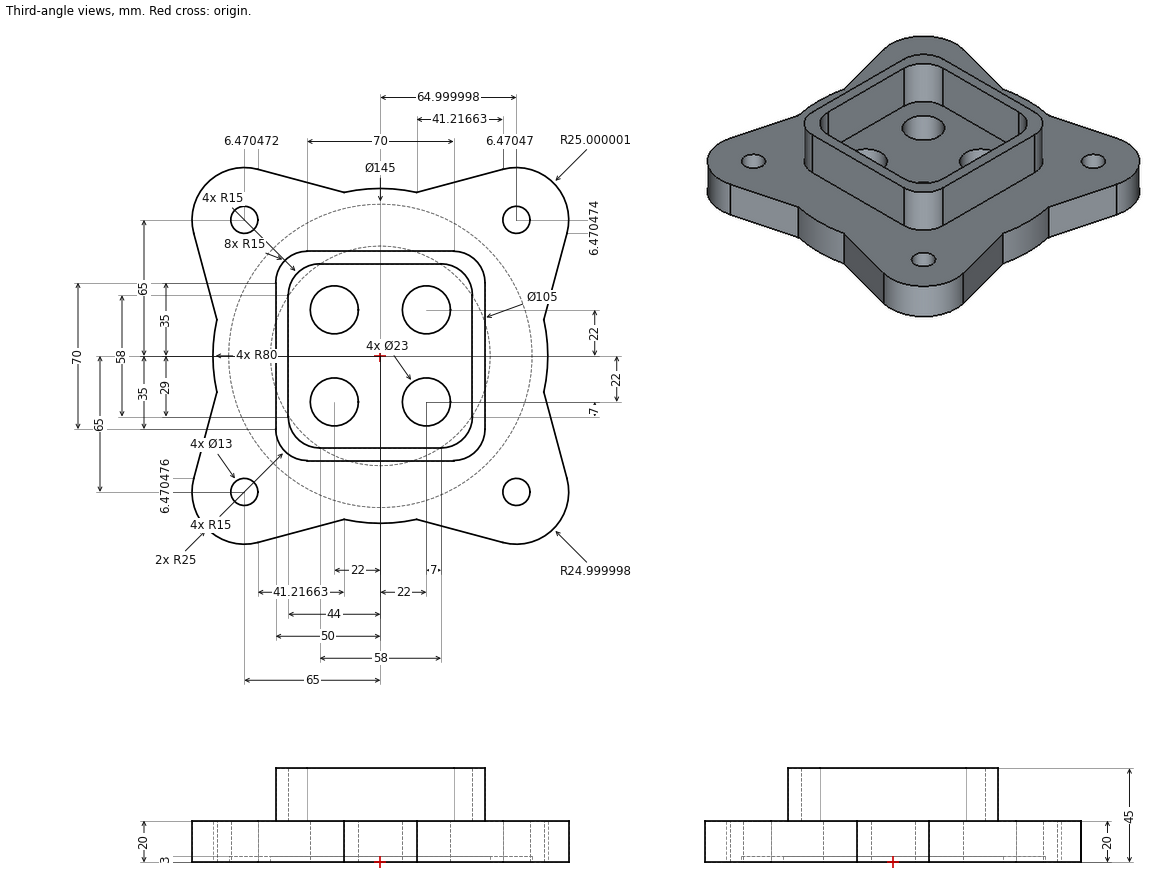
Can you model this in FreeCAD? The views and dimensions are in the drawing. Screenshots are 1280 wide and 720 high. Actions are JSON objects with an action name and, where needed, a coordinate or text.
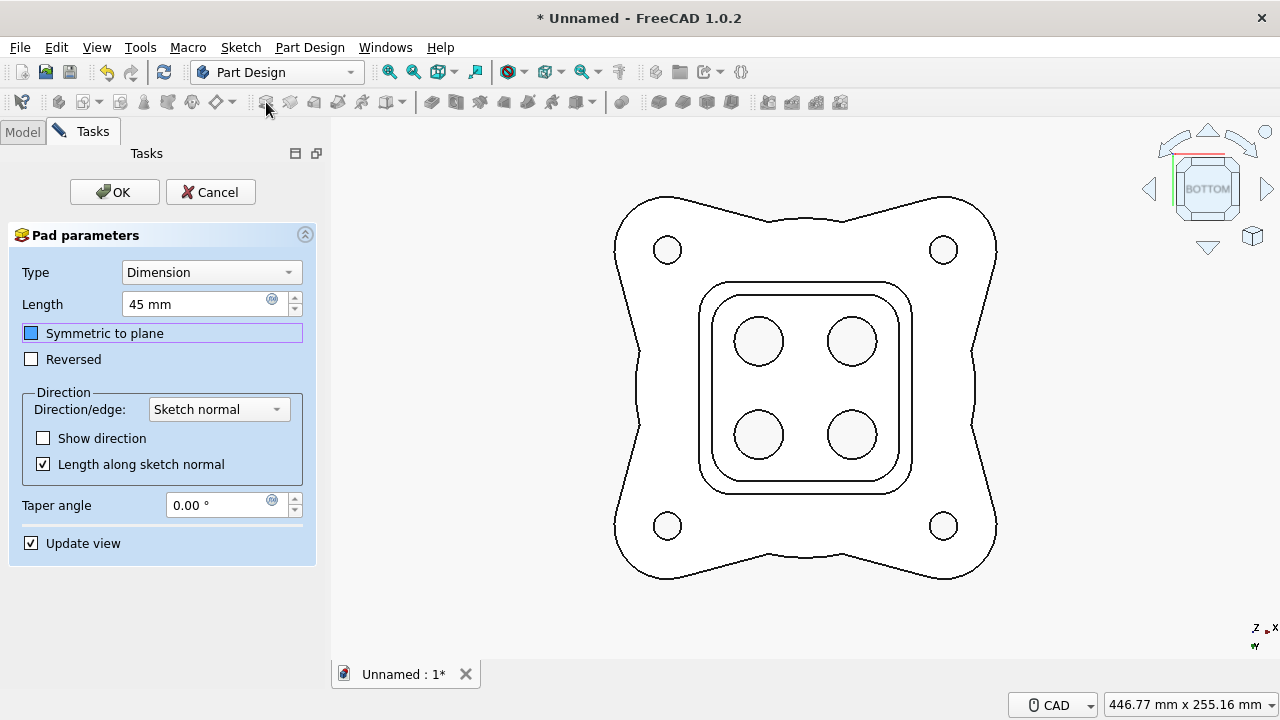
{"action": "left_click", "coordinate": [30, 359]}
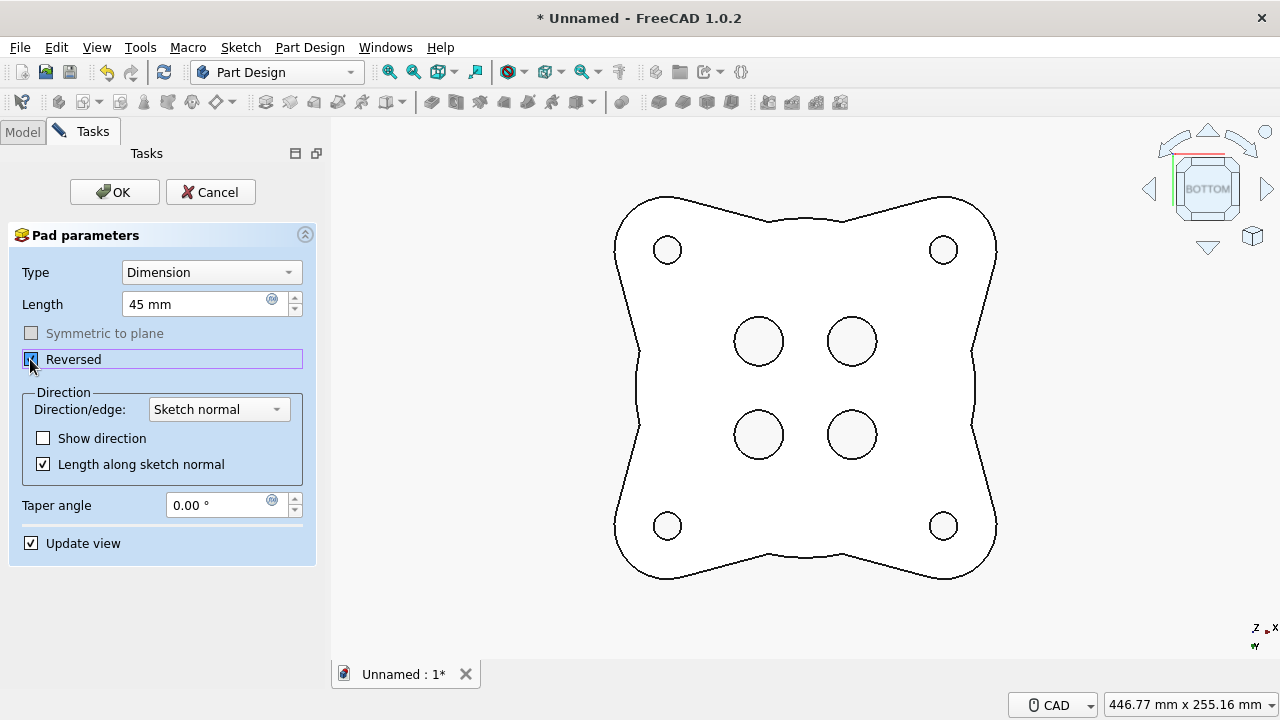
{"action": "left_click", "coordinate": [115, 192]}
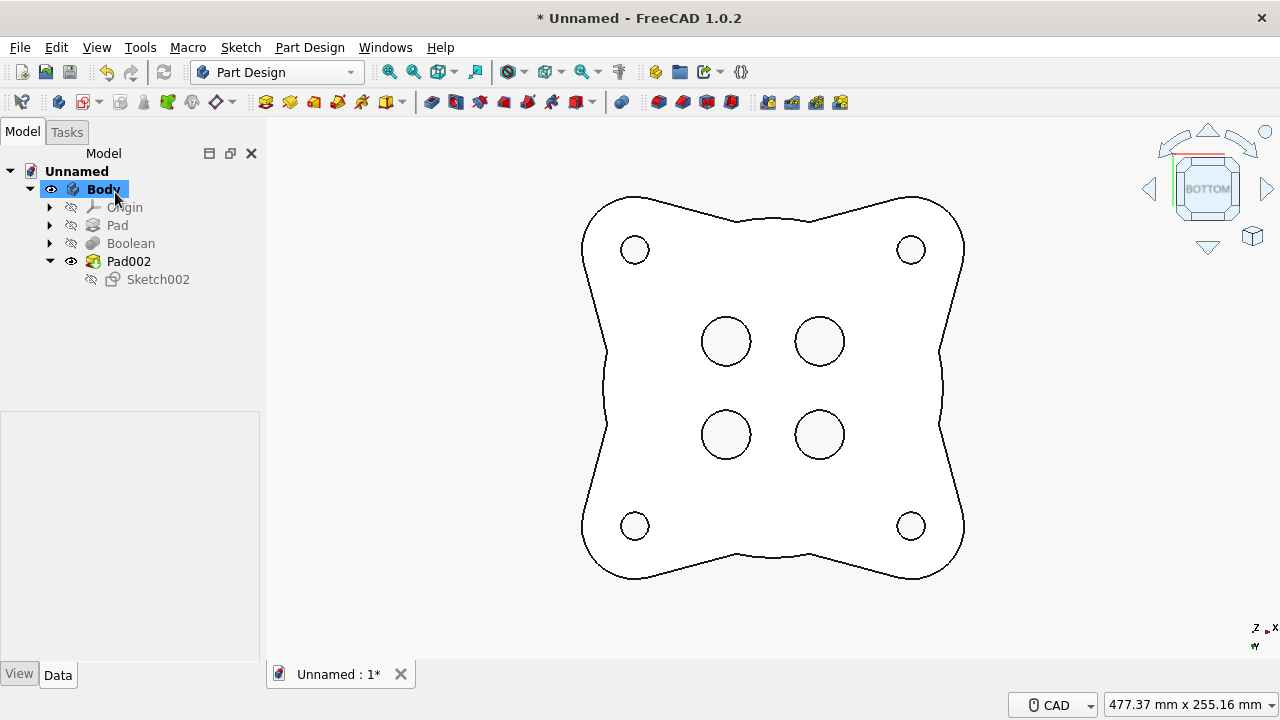
{"action": "left_click", "coordinate": [84, 102]}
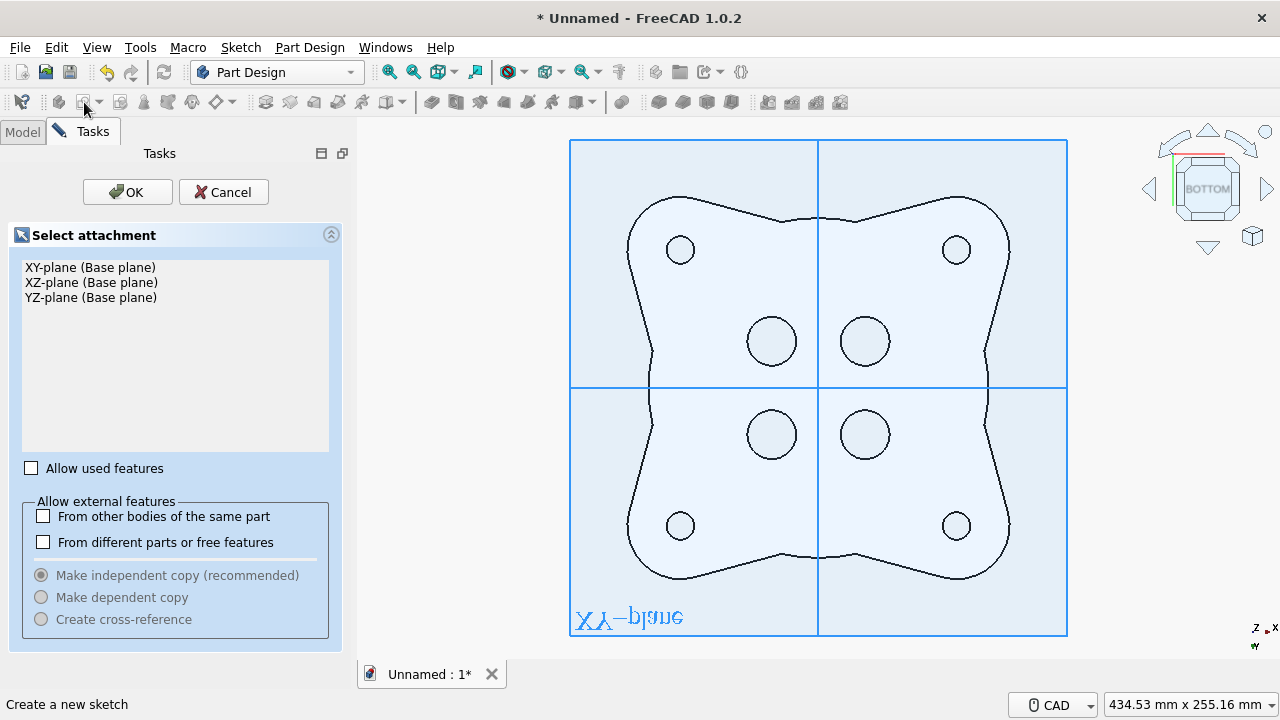
{"action": "left_click", "coordinate": [82, 268]}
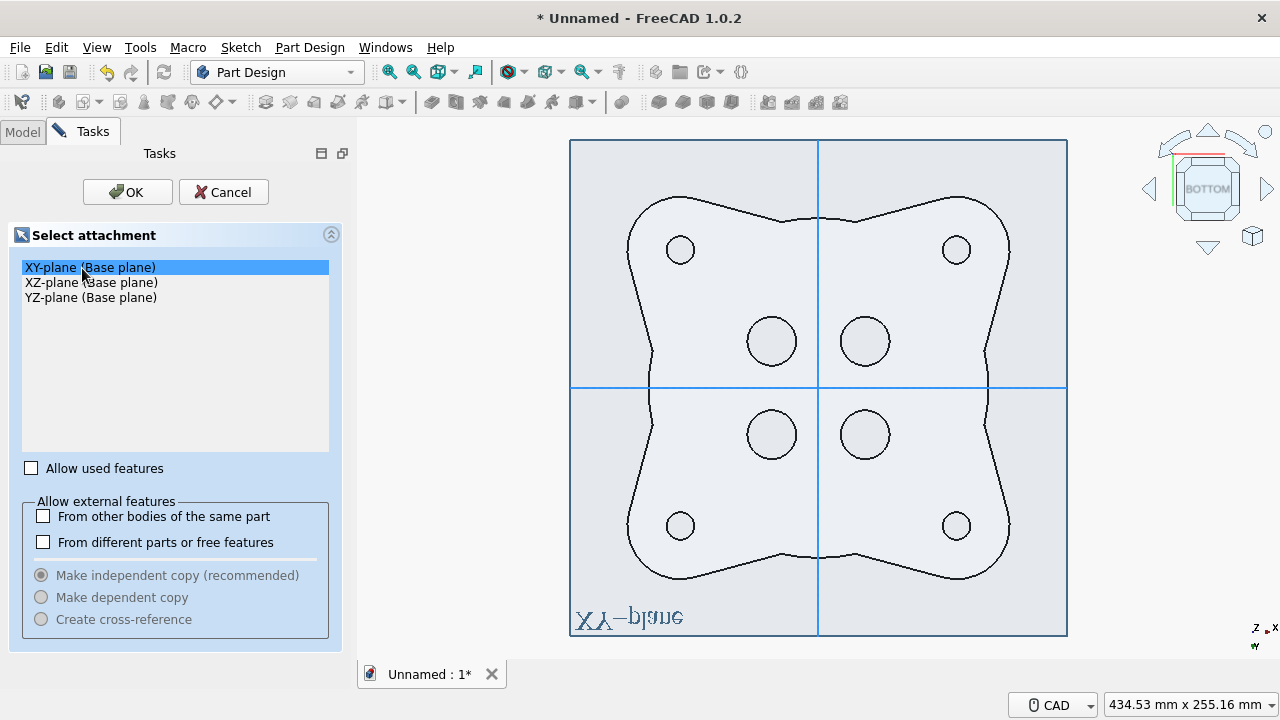
{"action": "left_click", "coordinate": [128, 192]}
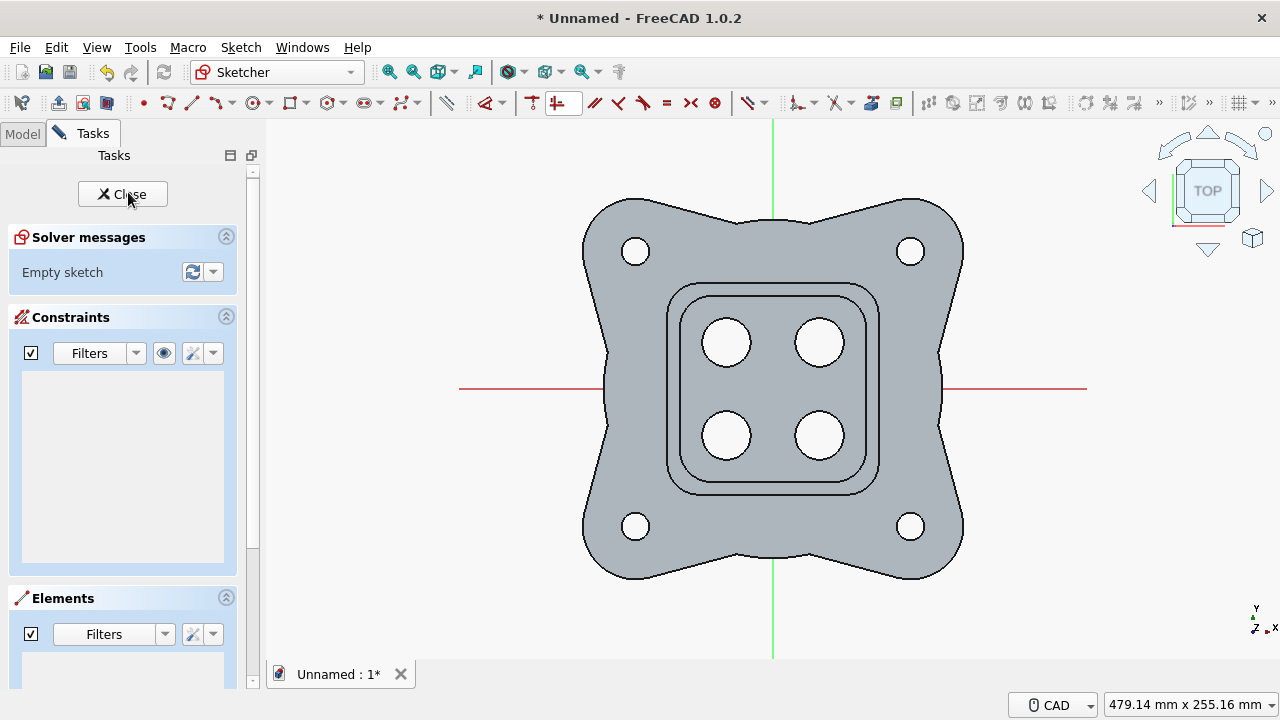
{"action": "left_click", "coordinate": [108, 104]}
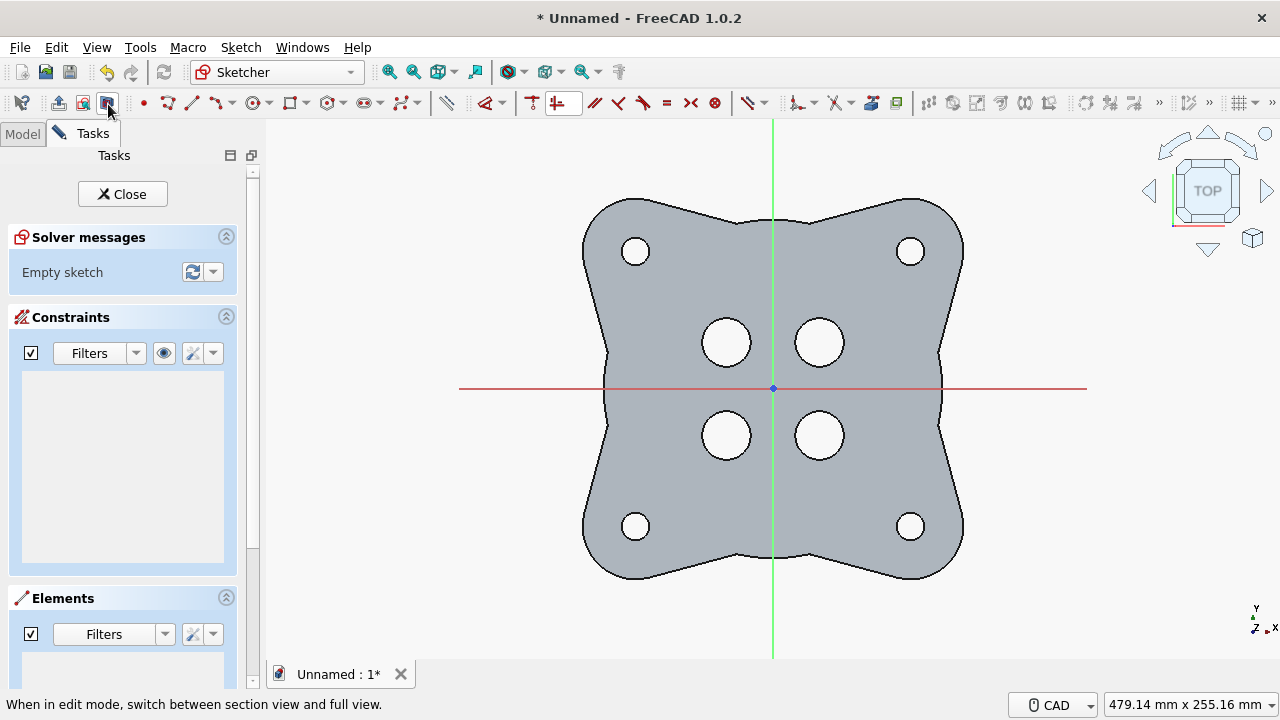
{"action": "left_click", "coordinate": [254, 104]}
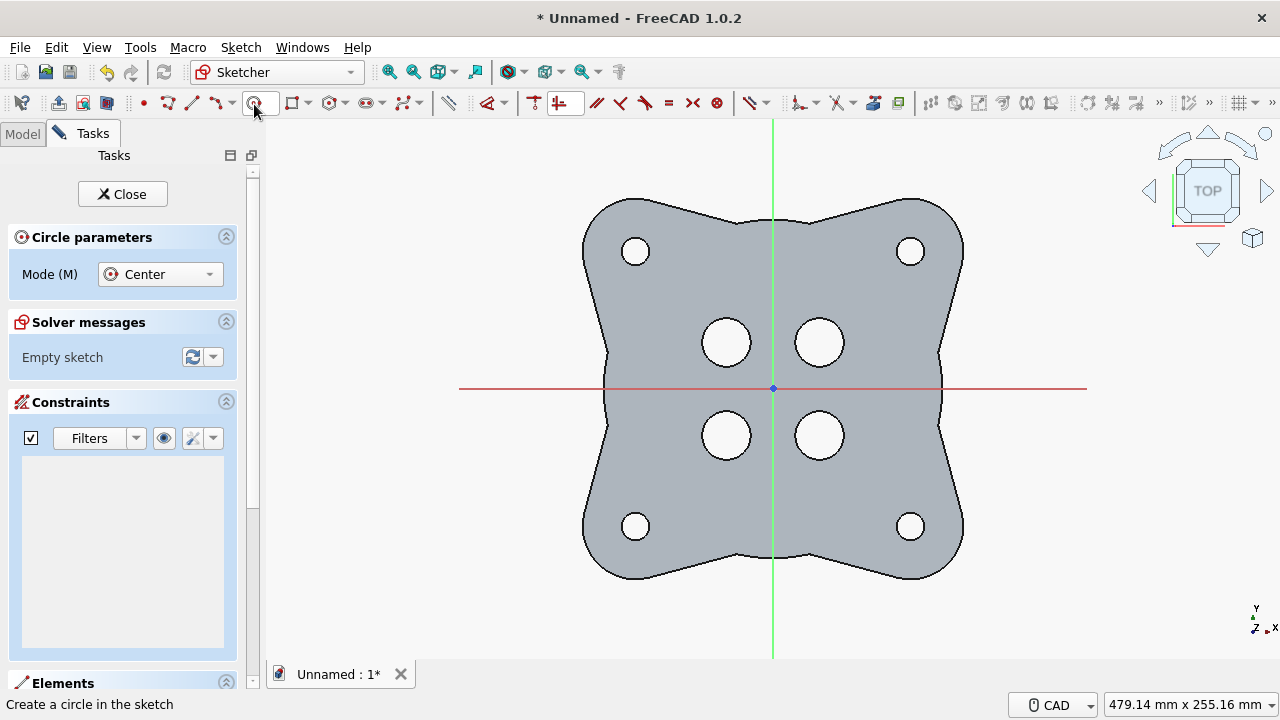
{"action": "left_click", "coordinate": [773, 389]}
{"action": "mouse_move", "coordinate": [881, 281]}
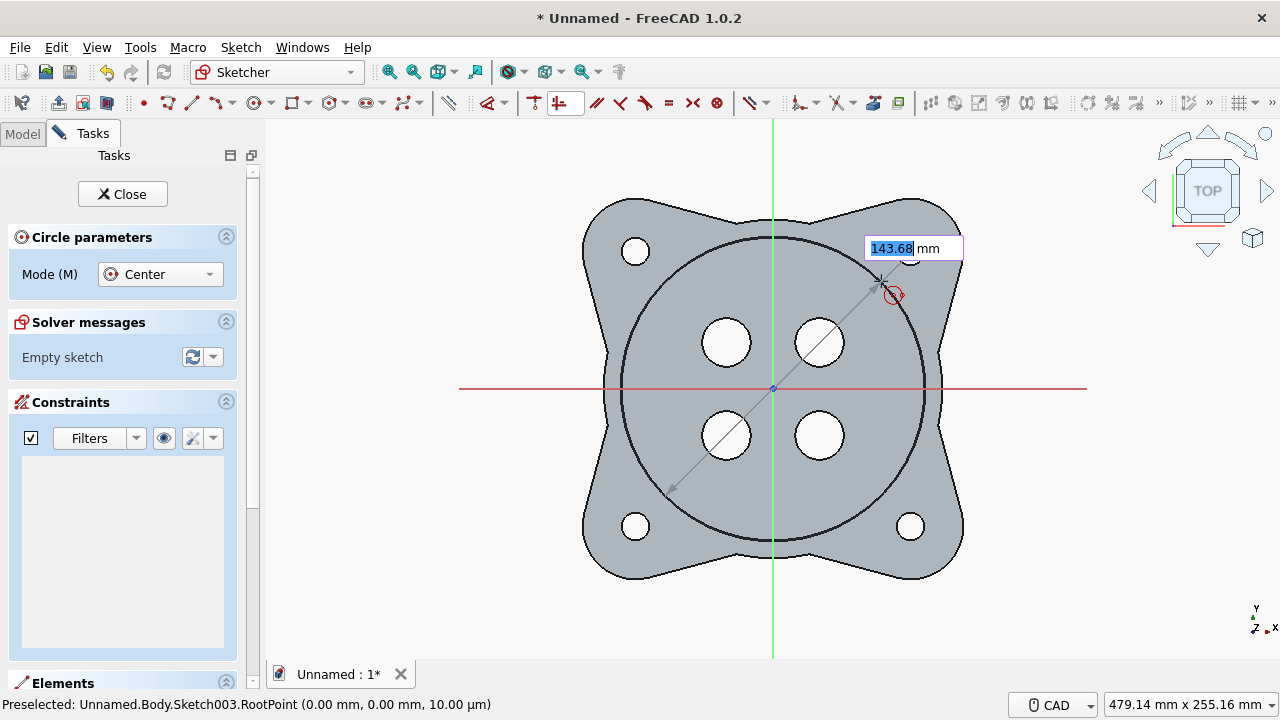
{"action": "type", "text": "145"}
{"action": "key", "text": "Return"}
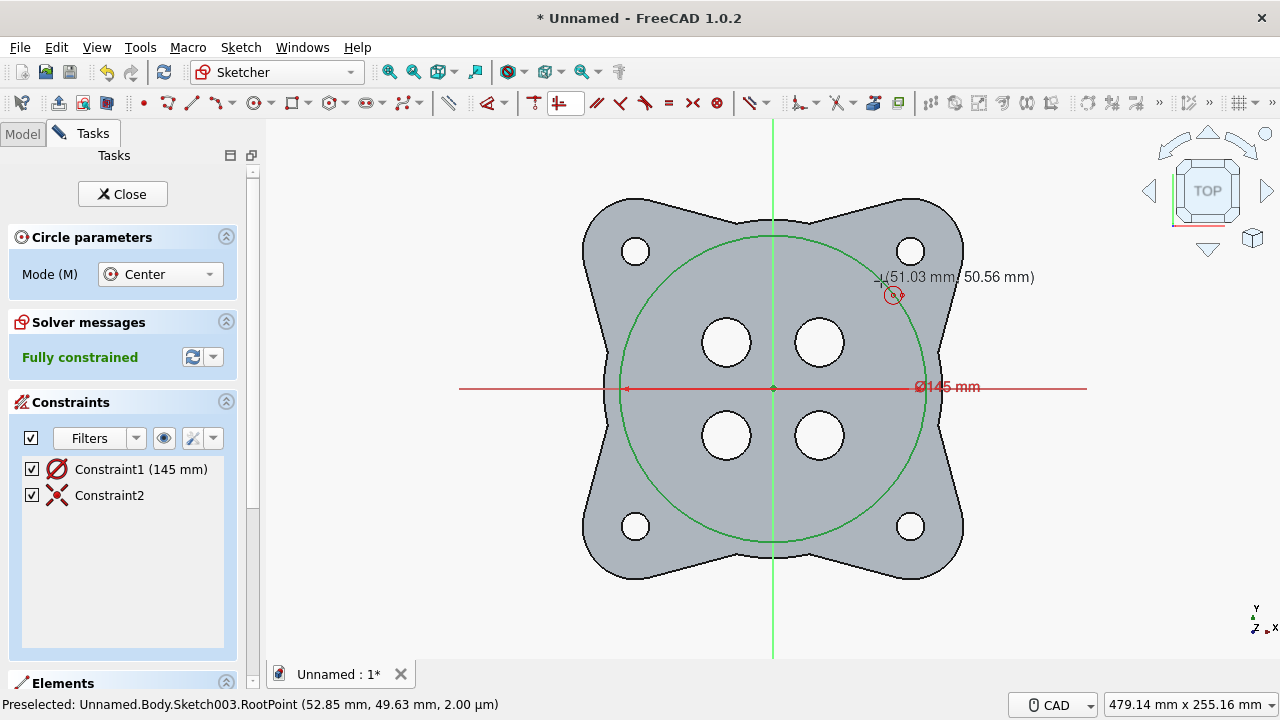
{"action": "left_click", "coordinate": [773, 389]}
{"action": "mouse_move", "coordinate": [852, 310]}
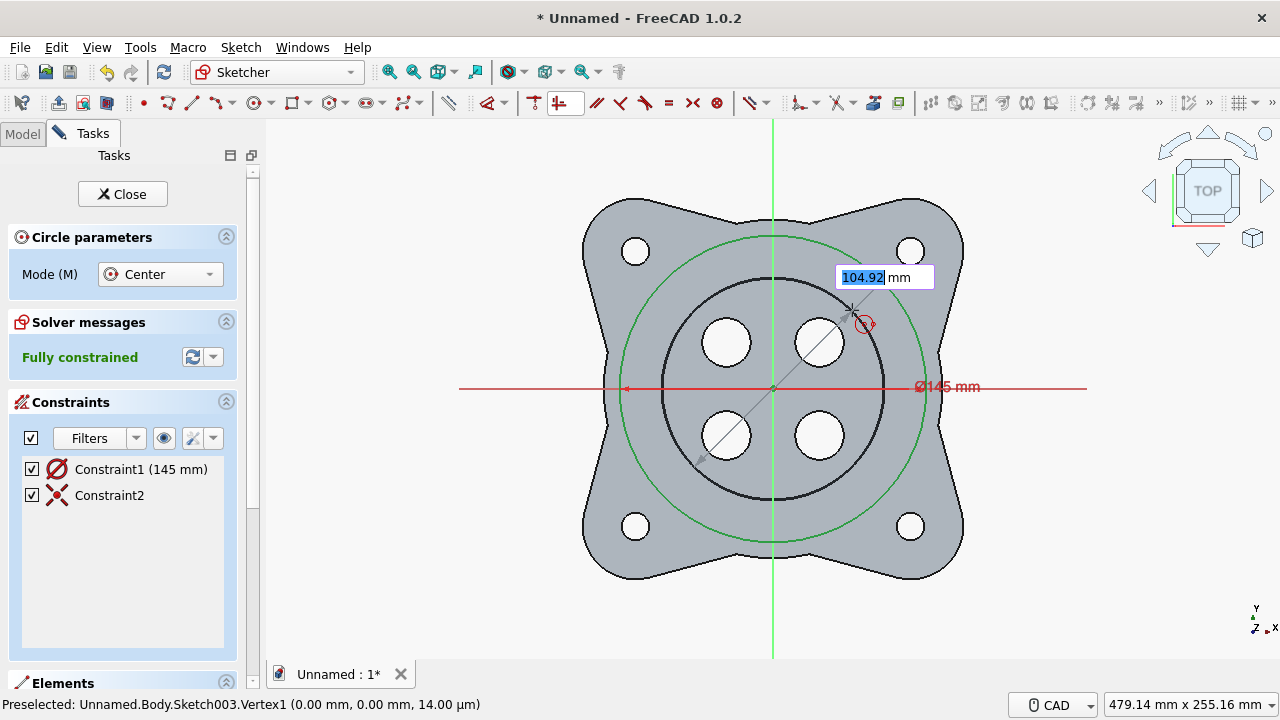
{"action": "type", "text": "105"}
{"action": "key", "text": "Return"}
{"action": "key", "text": "Escape"}